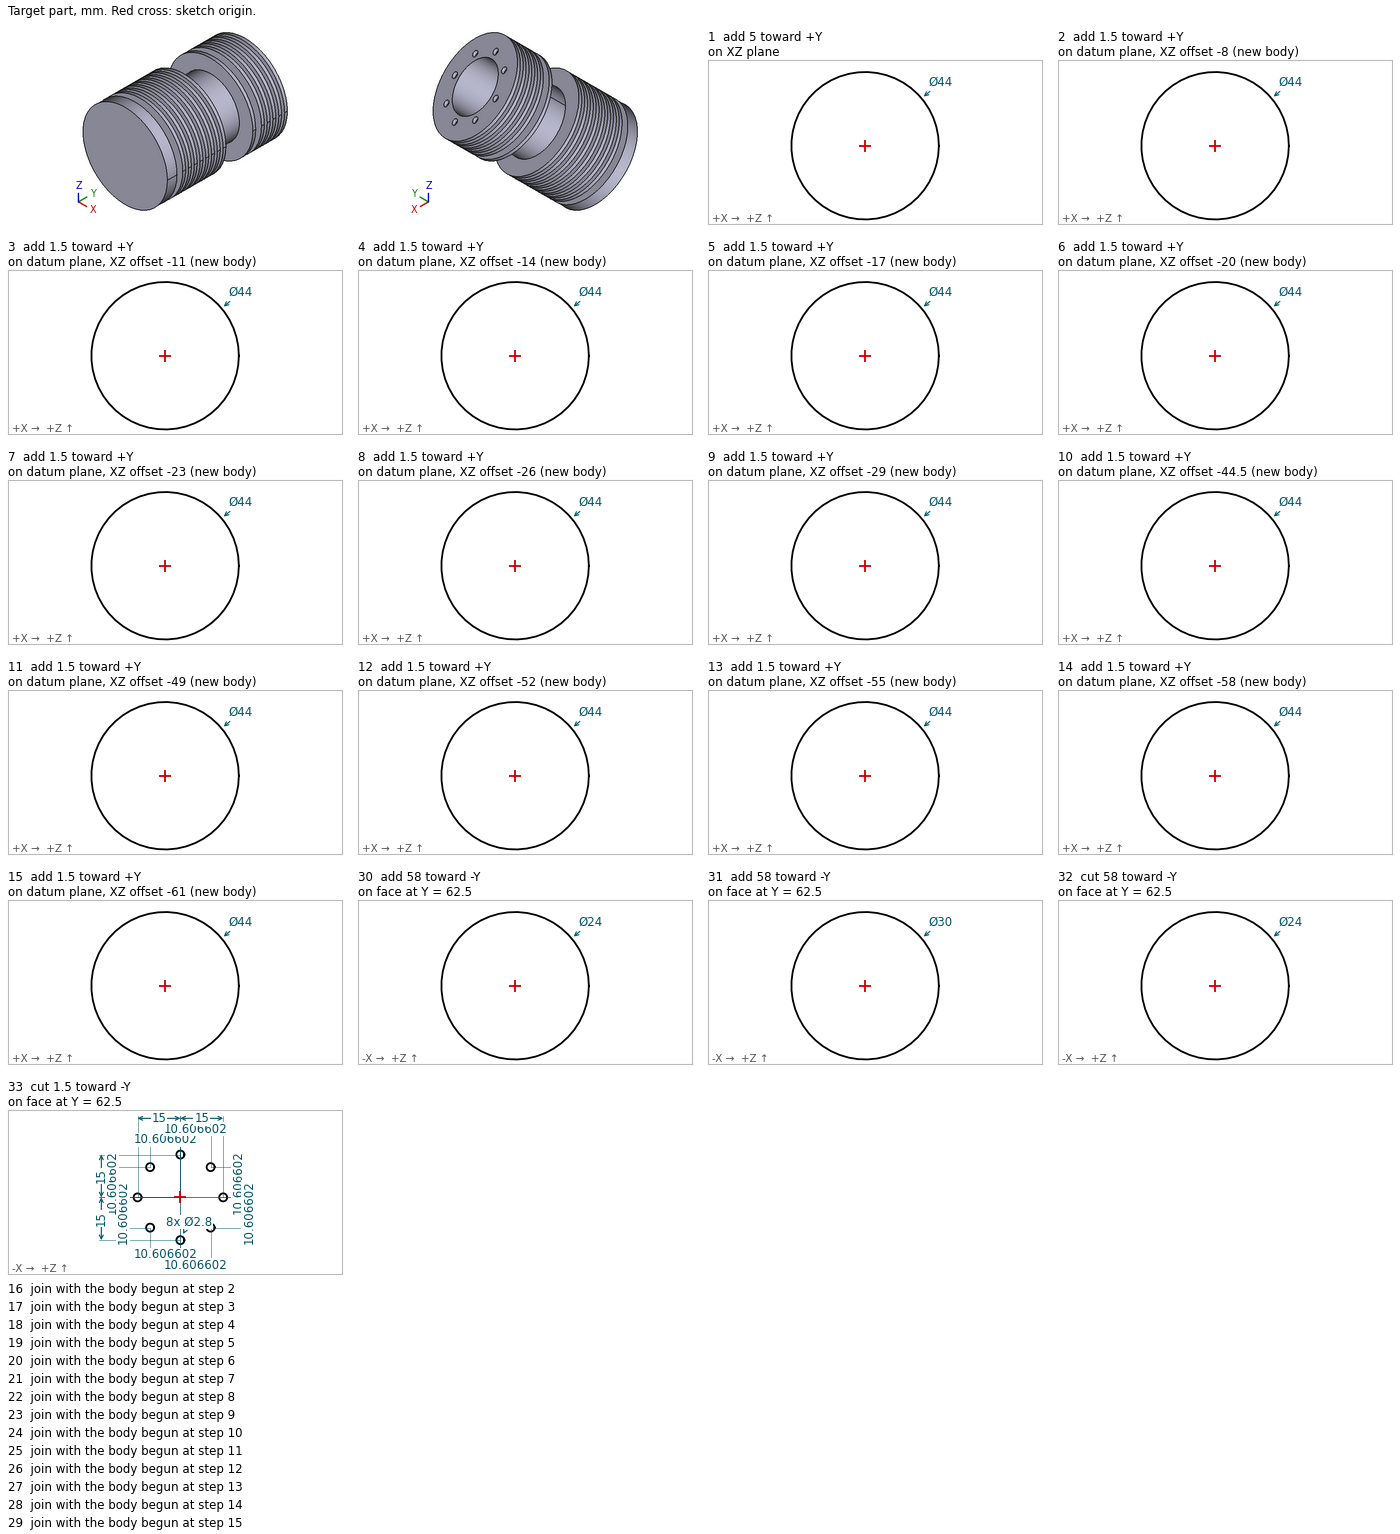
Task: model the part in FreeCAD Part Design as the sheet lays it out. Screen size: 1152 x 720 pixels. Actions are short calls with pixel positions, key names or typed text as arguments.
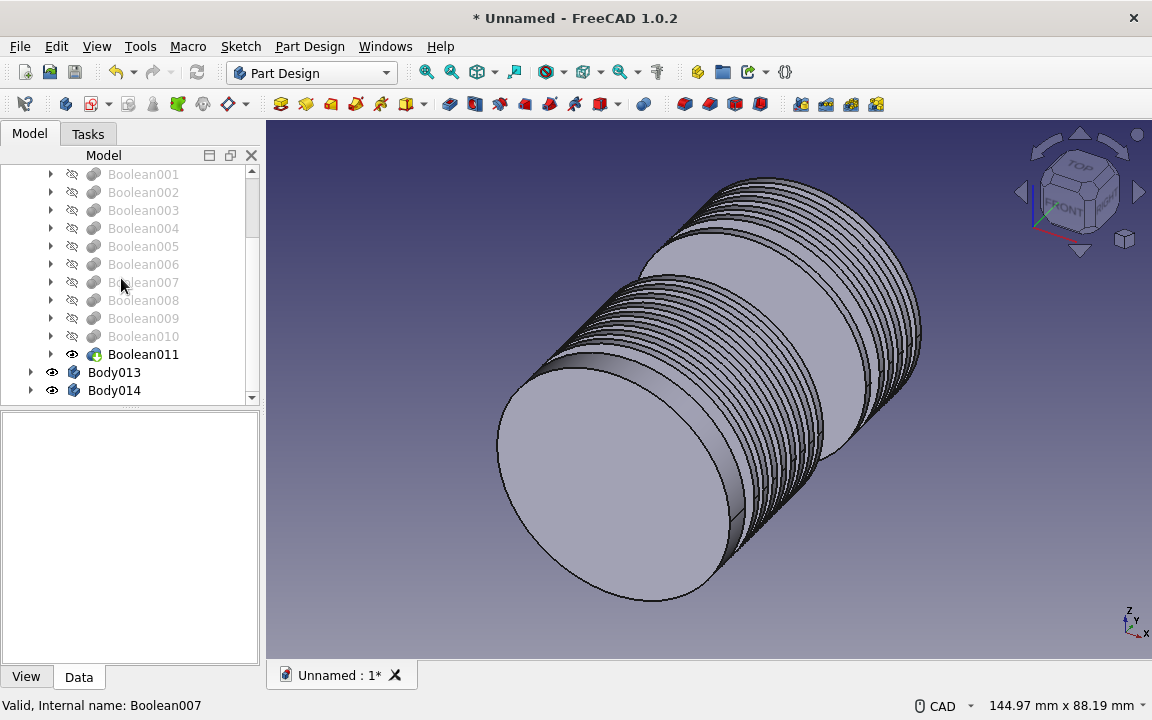
click(97, 372)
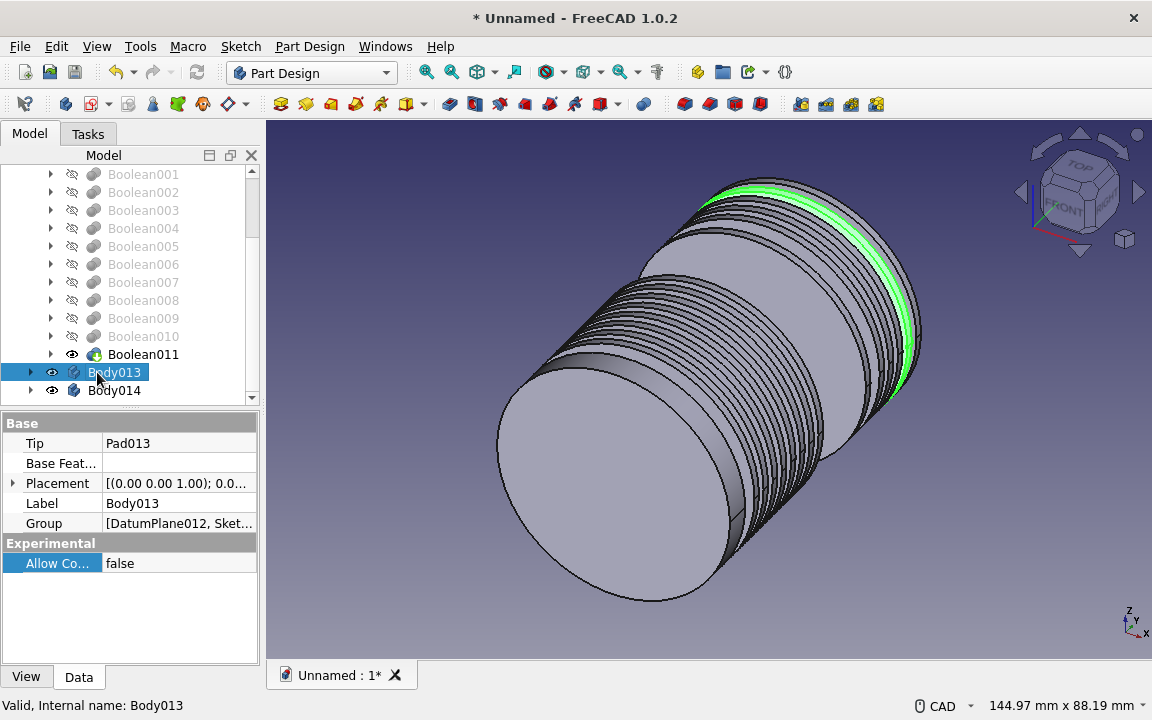
click(644, 104)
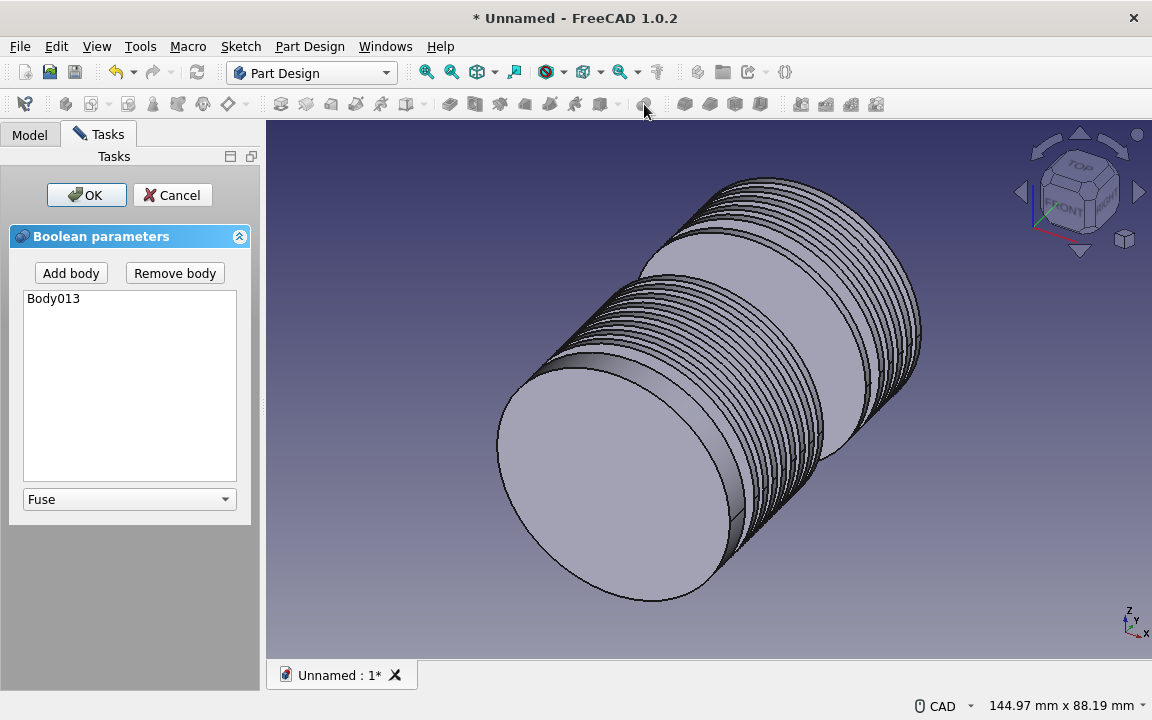
click(87, 195)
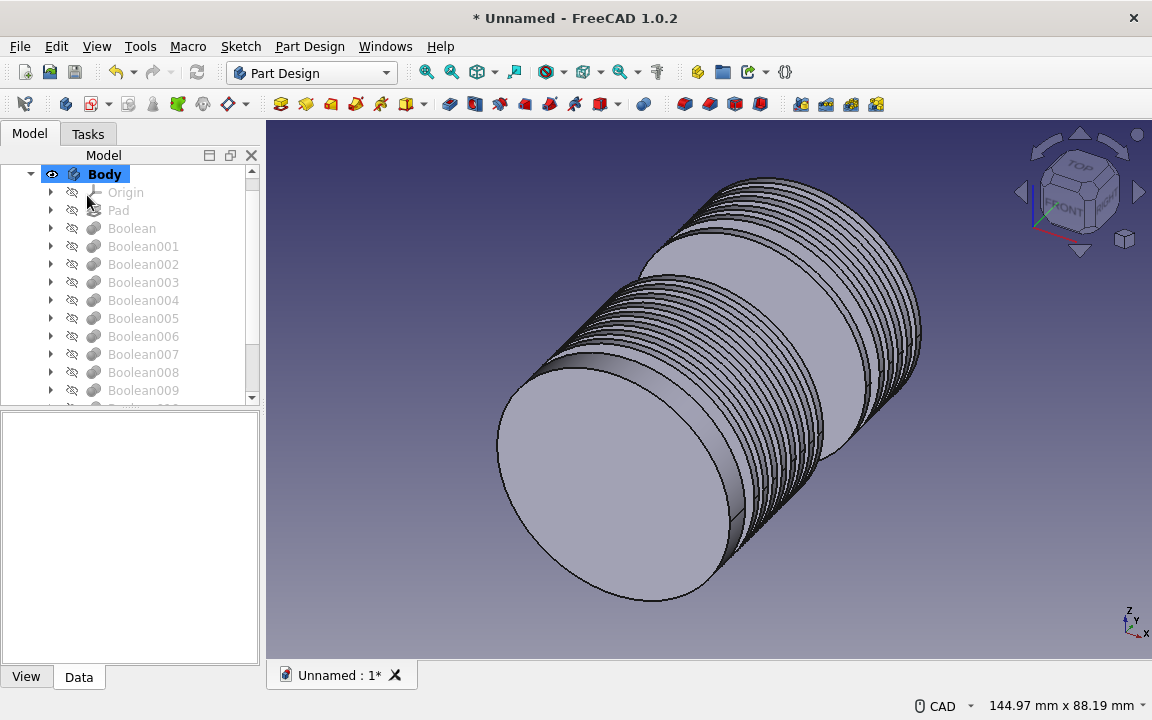
scroll(121, 278, down, 3)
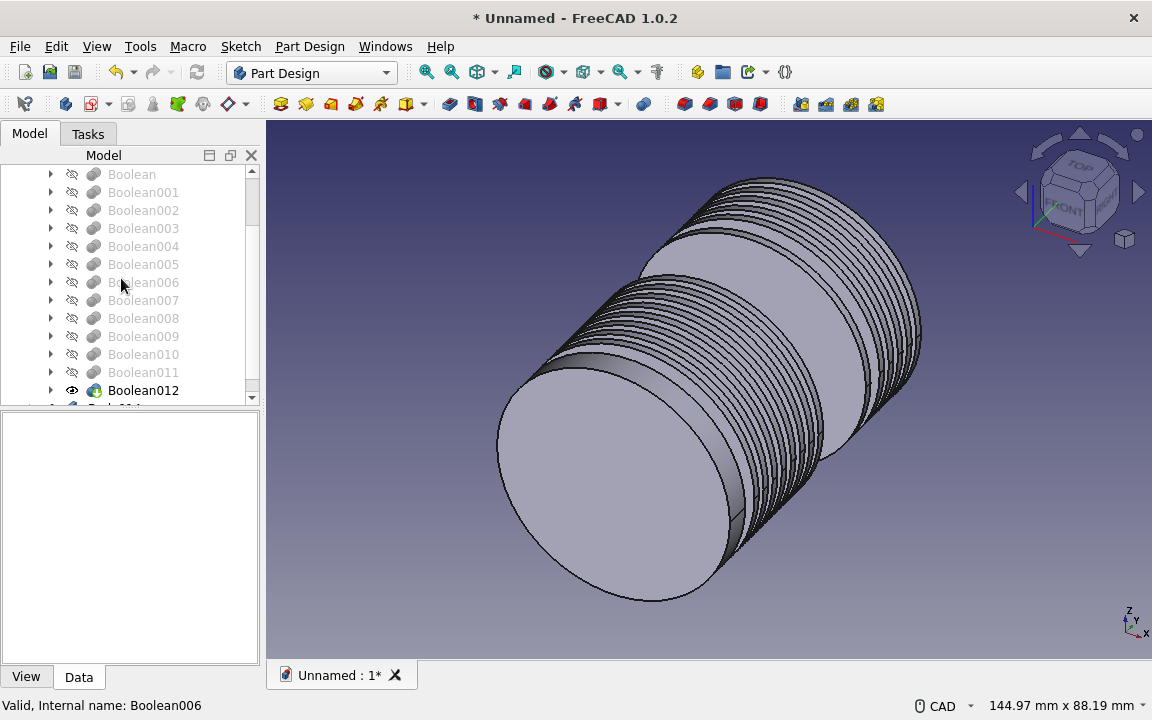
click(97, 390)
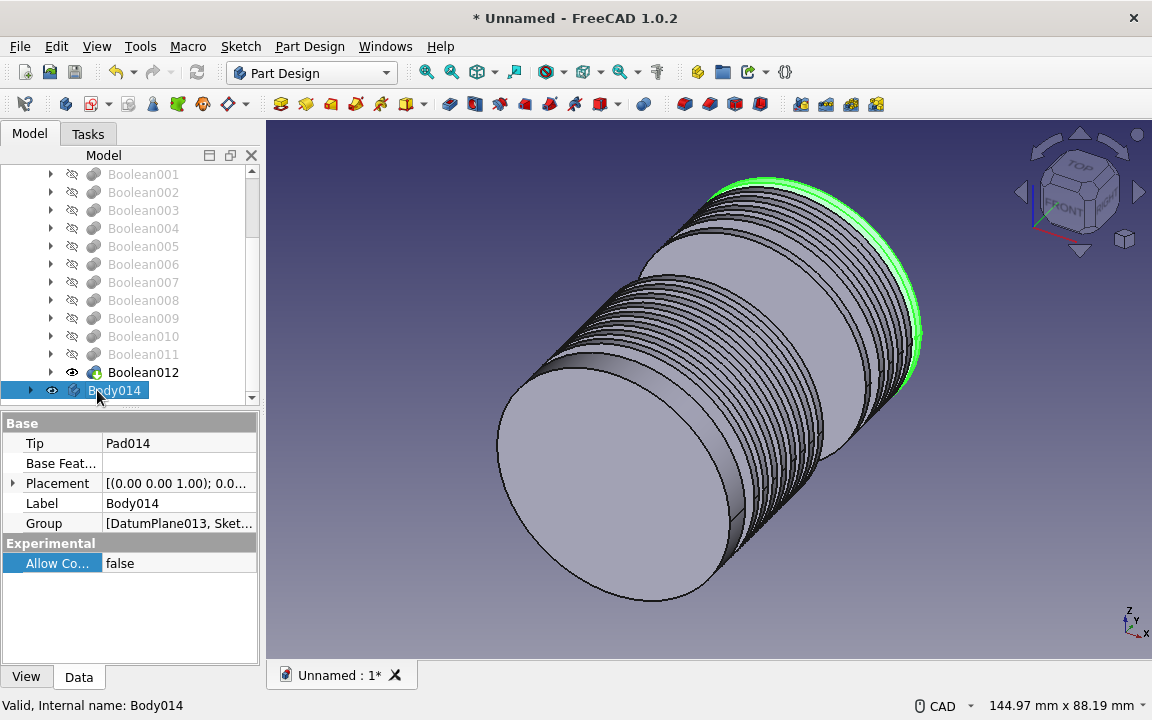
click(644, 104)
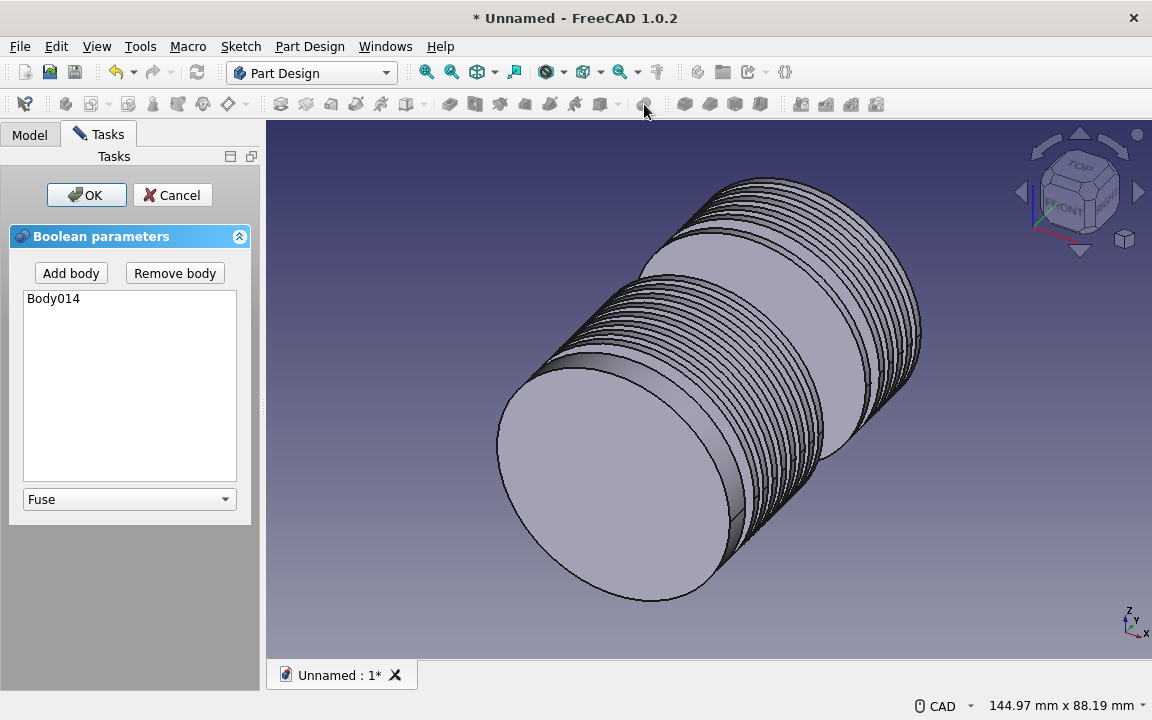
click(87, 195)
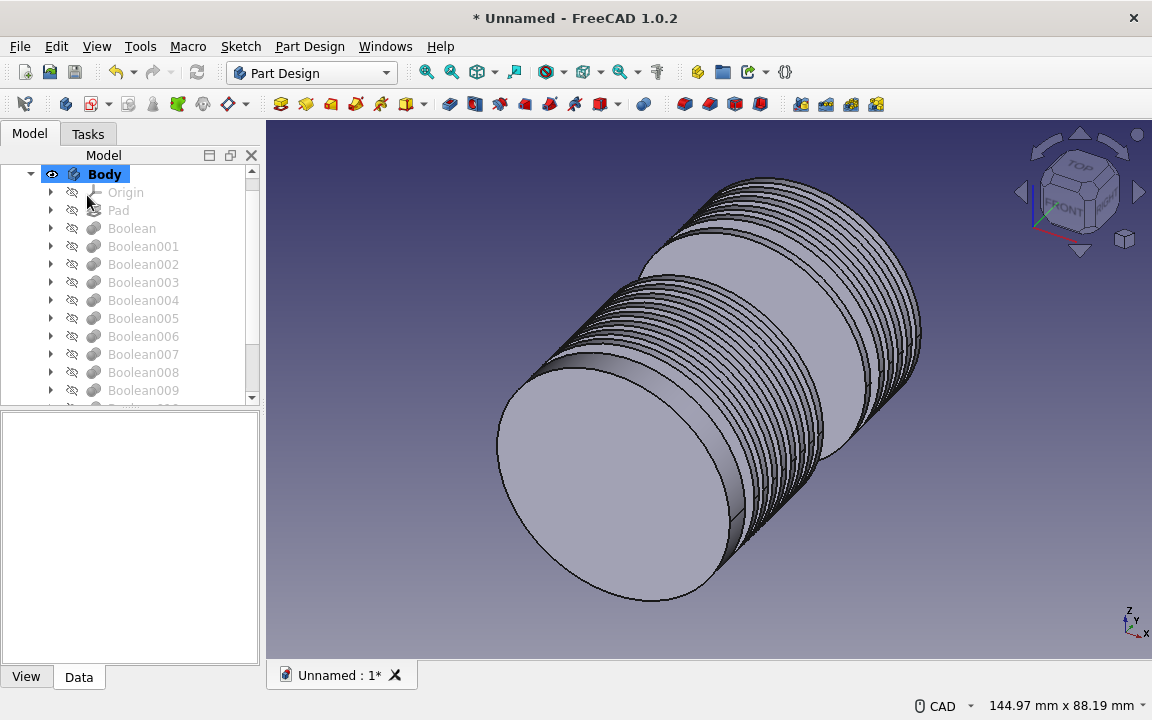
key(4)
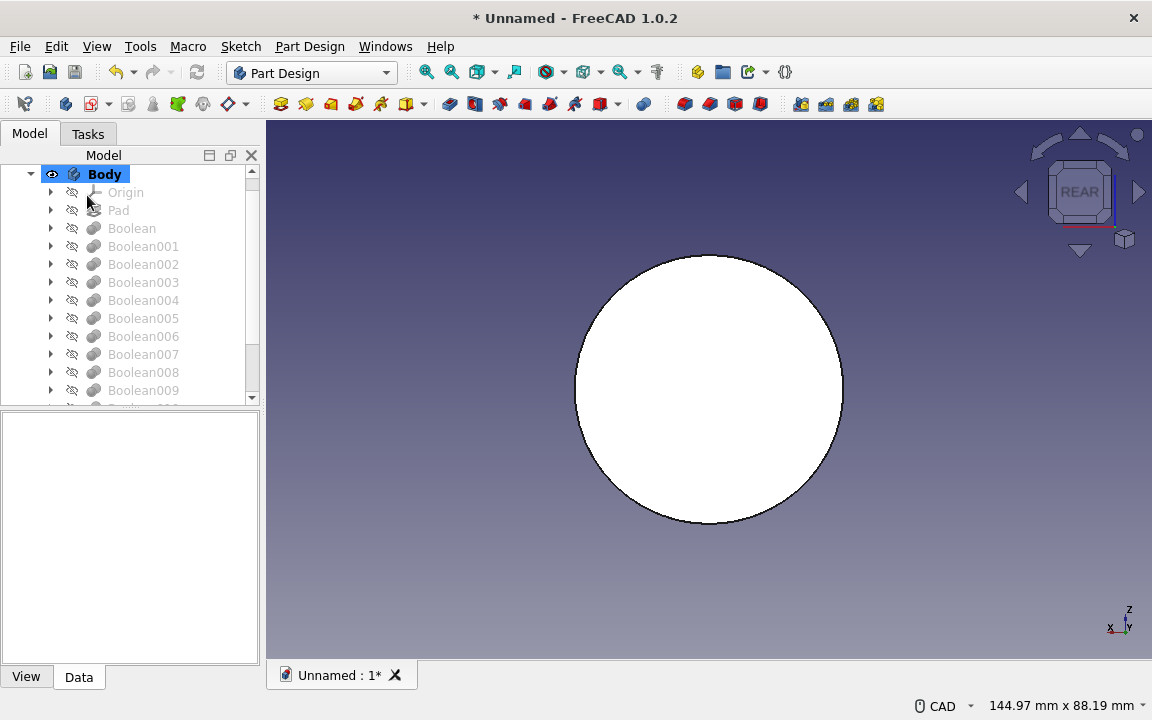
click(709, 389)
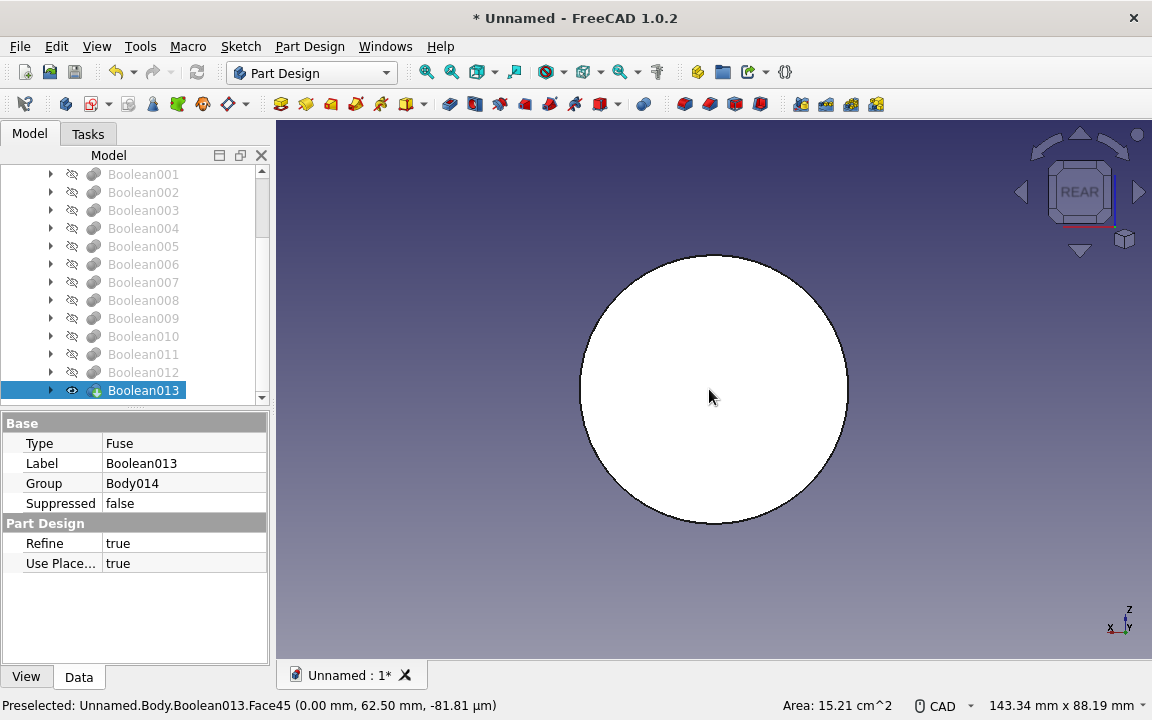
click(90, 104)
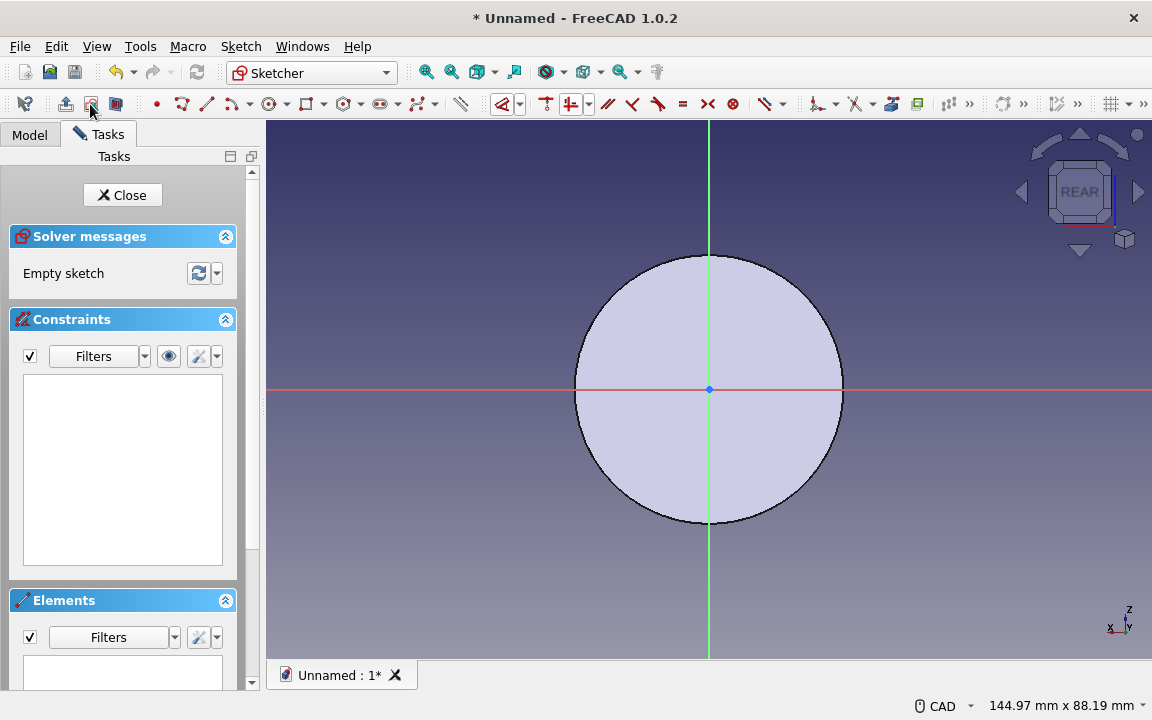
scroll(765, 390, up, 4)